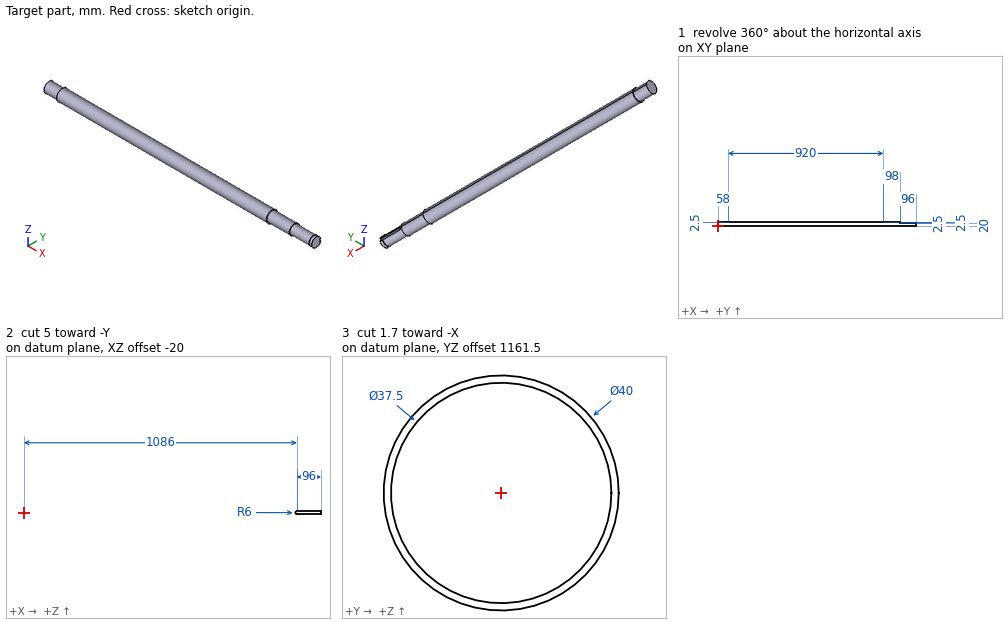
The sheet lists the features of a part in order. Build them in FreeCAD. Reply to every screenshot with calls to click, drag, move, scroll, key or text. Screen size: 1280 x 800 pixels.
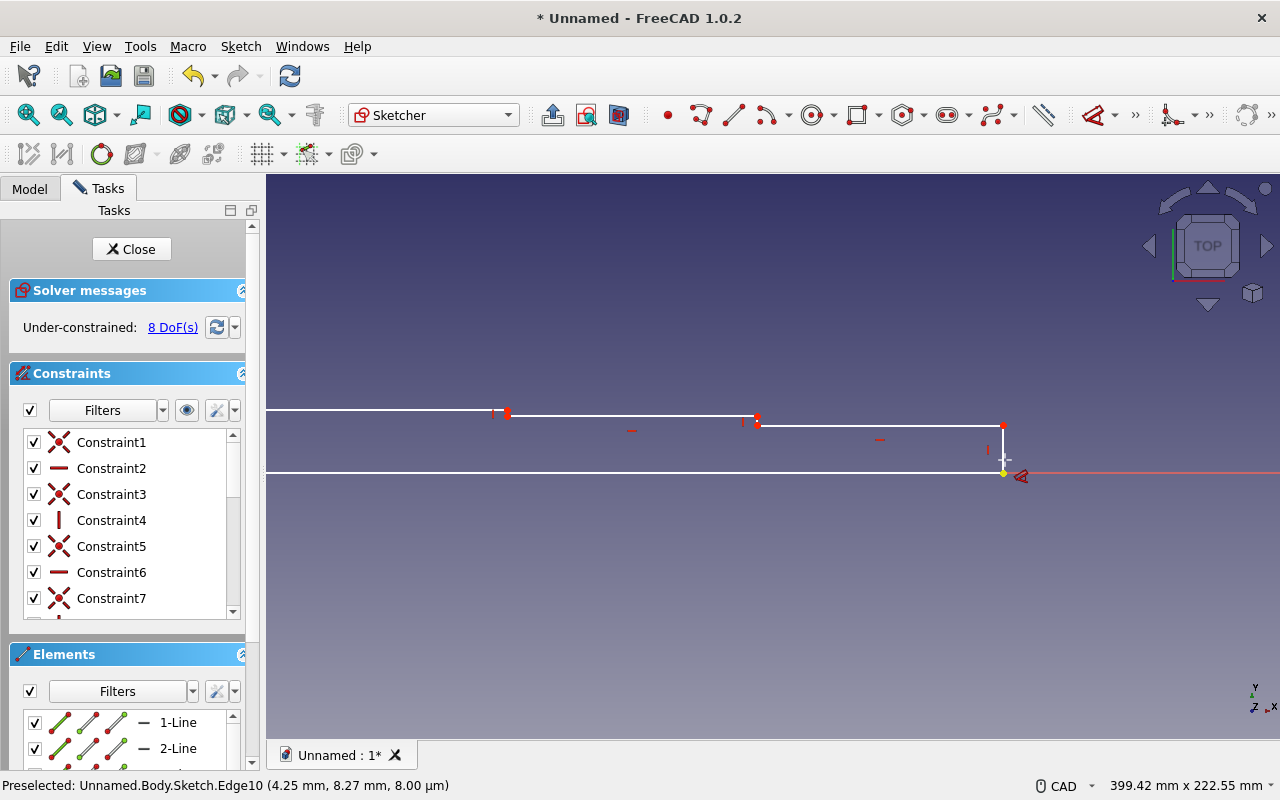
click(1003, 459)
click(1037, 449)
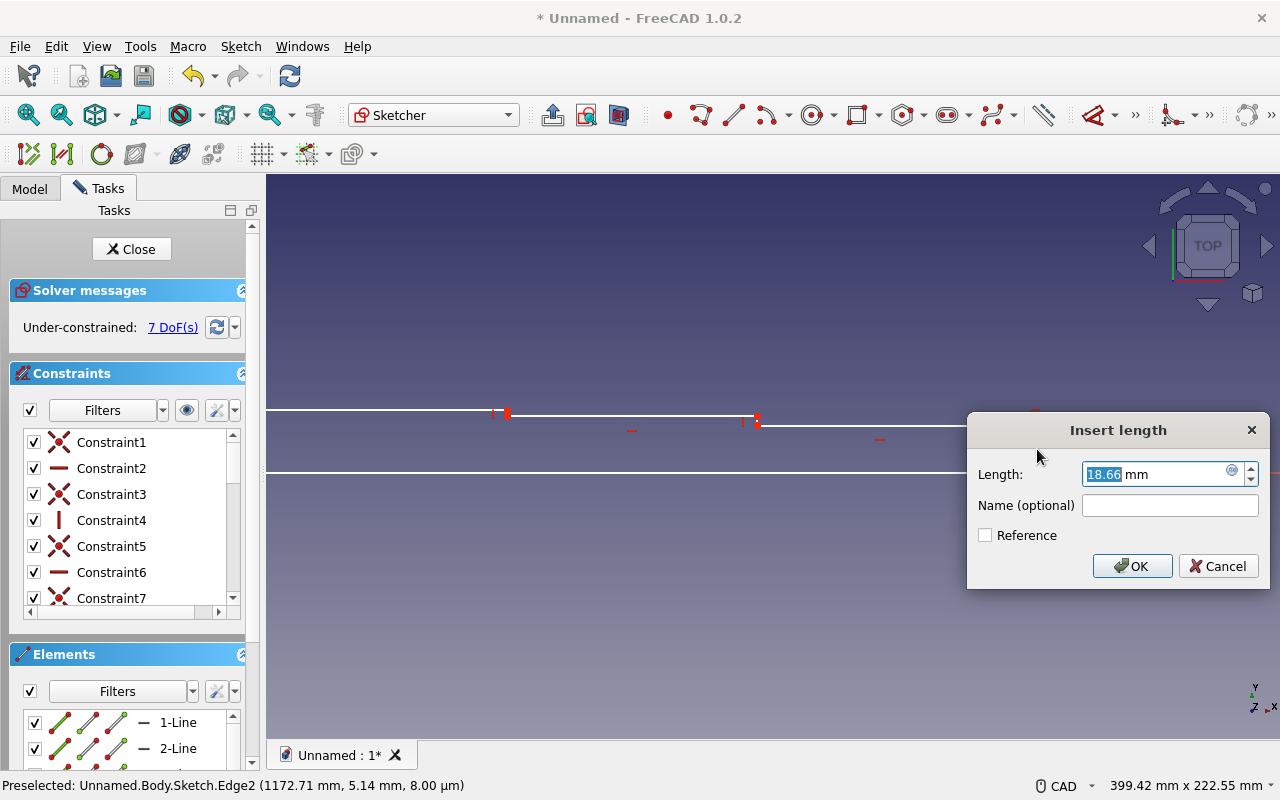
text(20)
key(Return)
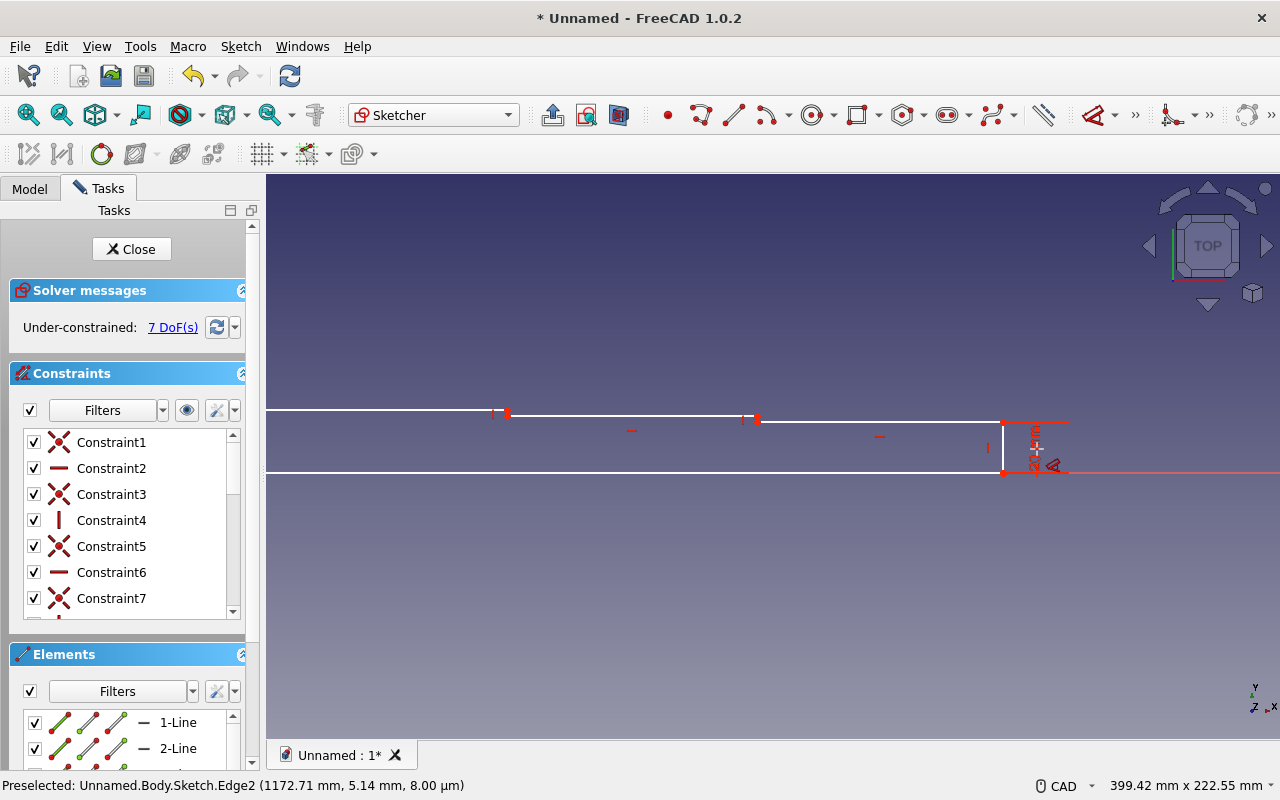
scroll(1006, 460, down, 8)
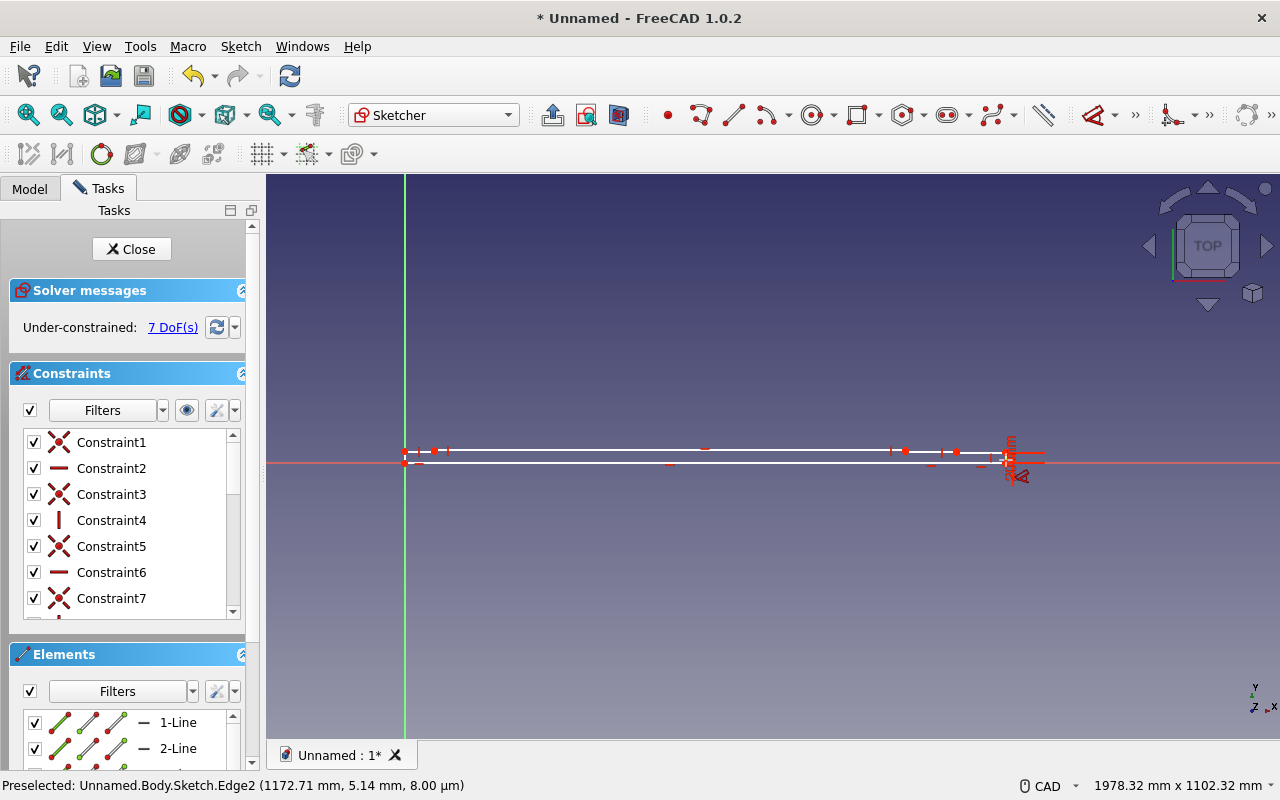
scroll(991, 453, up, 2)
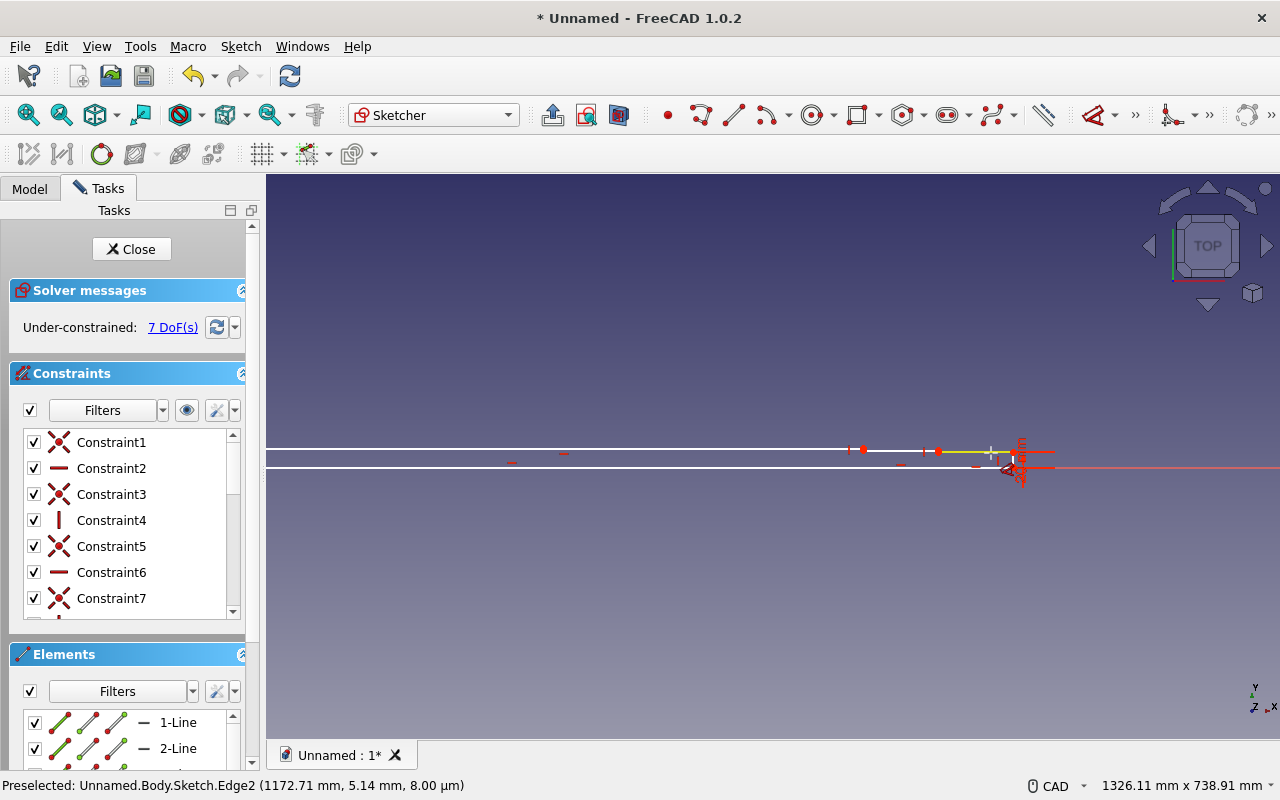
click(991, 452)
click(976, 418)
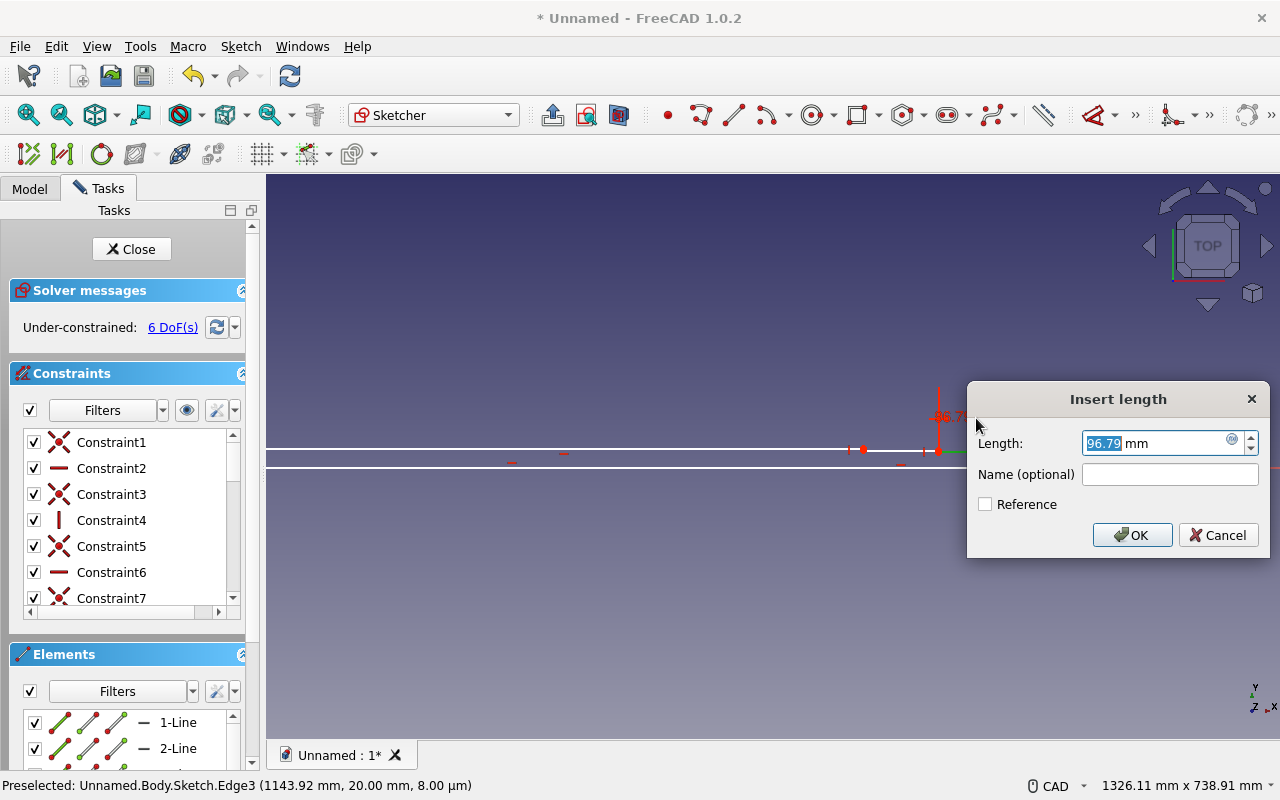
text(96)
key(Return)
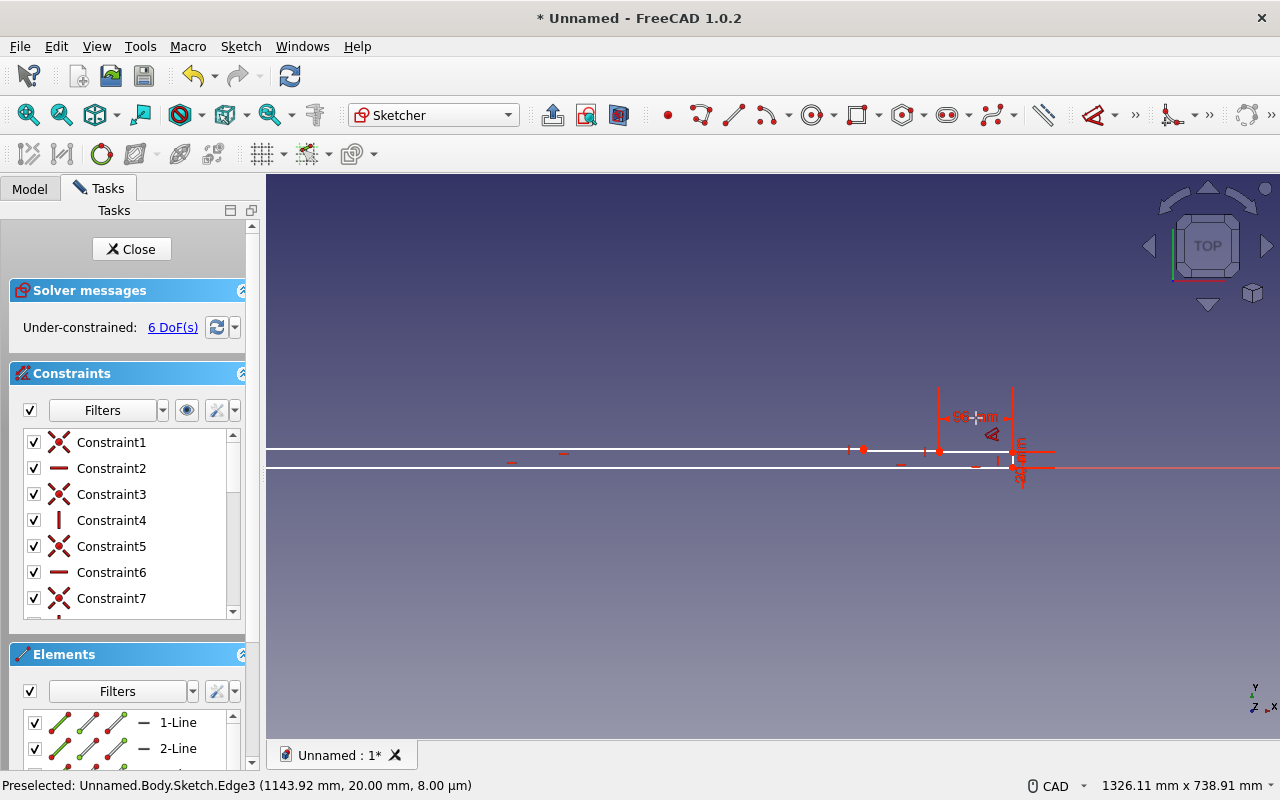
click(917, 451)
click(902, 417)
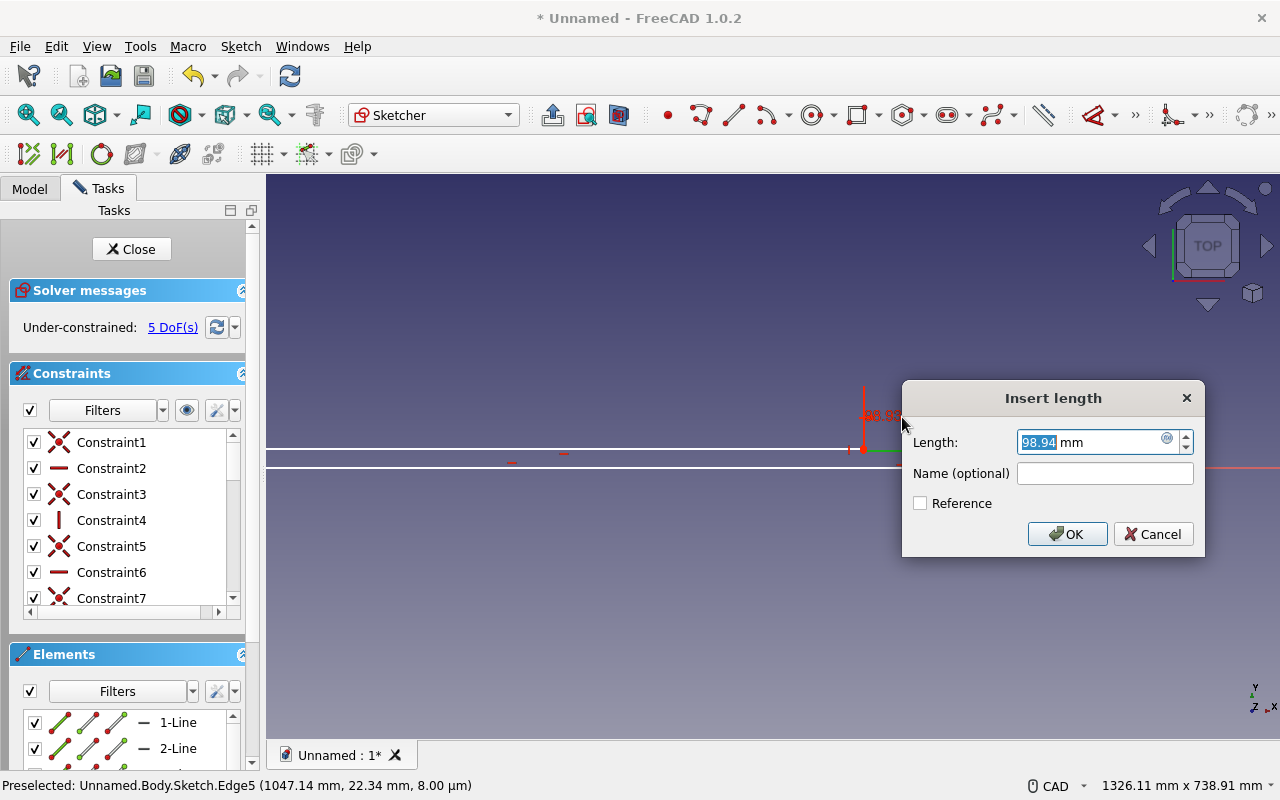
text(98)
key(Return)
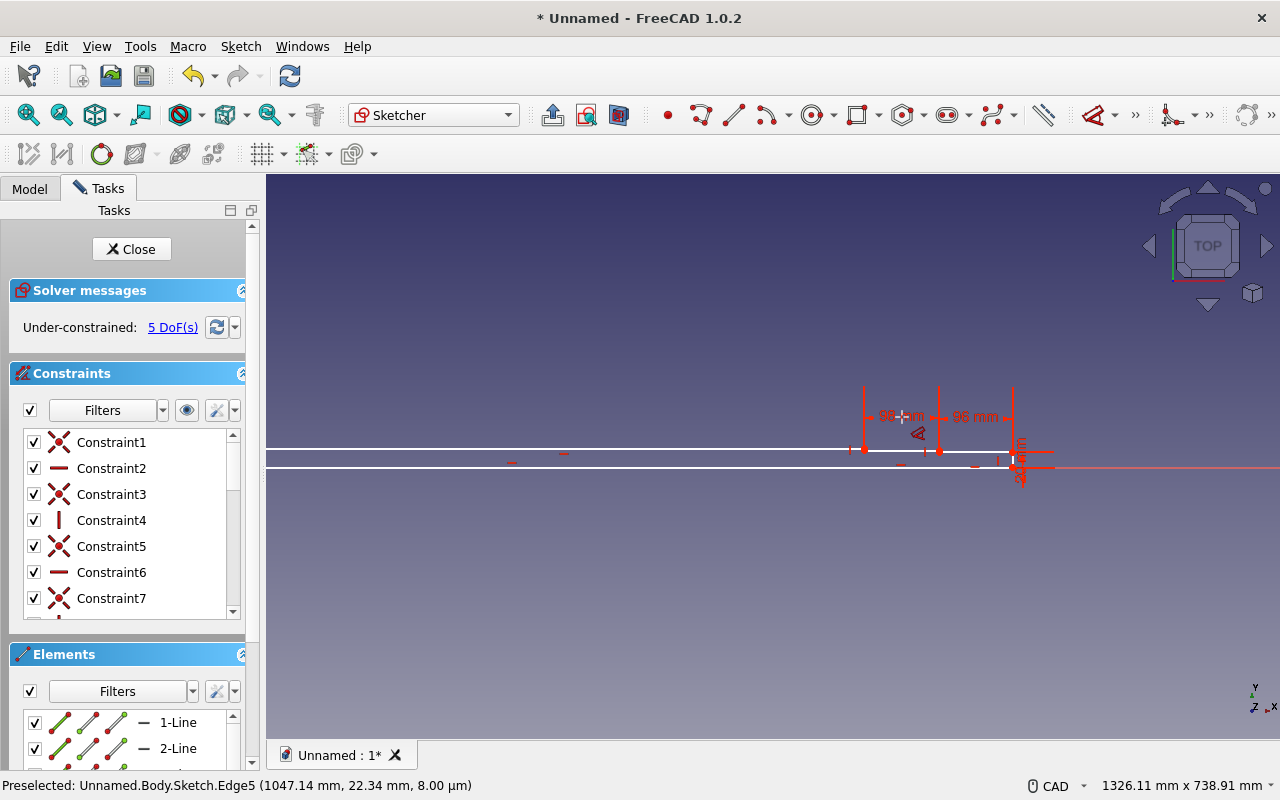
scroll(989, 453, down, 2)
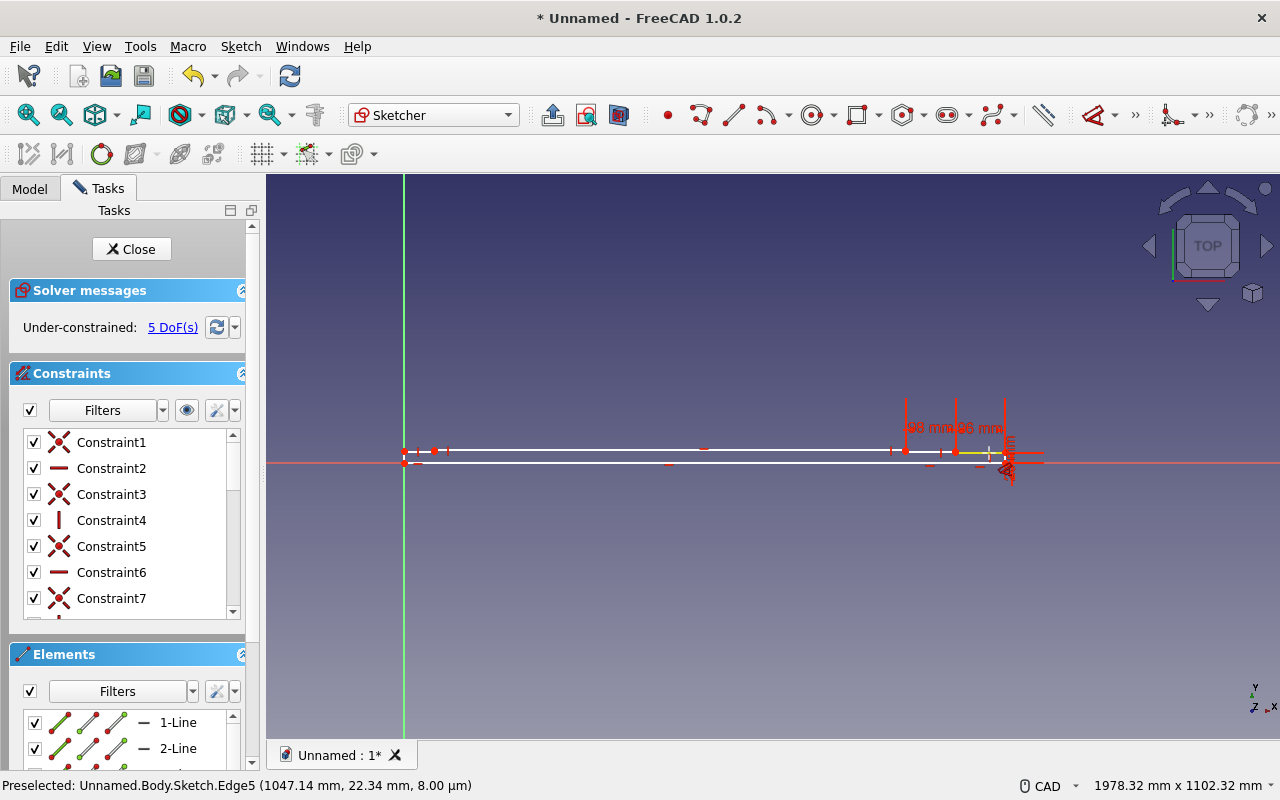
scroll(425, 452, up, 3)